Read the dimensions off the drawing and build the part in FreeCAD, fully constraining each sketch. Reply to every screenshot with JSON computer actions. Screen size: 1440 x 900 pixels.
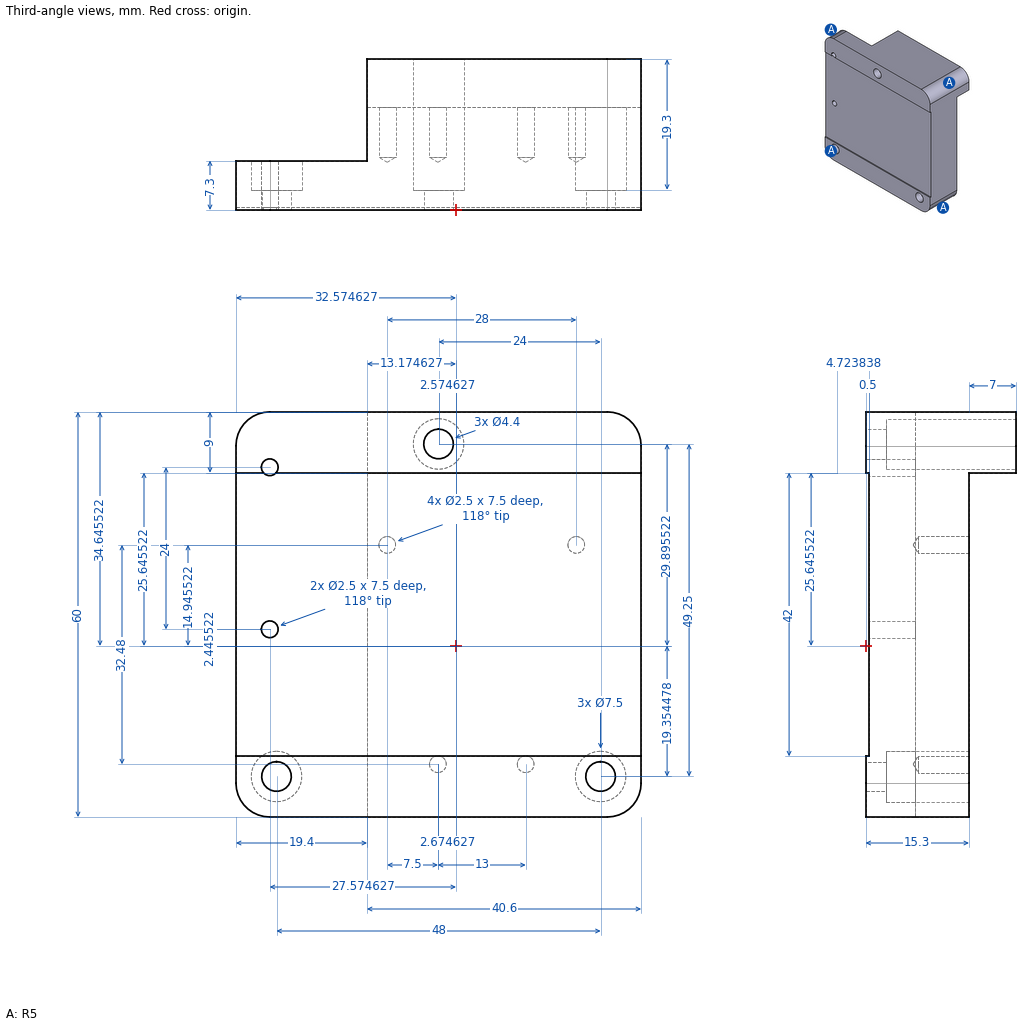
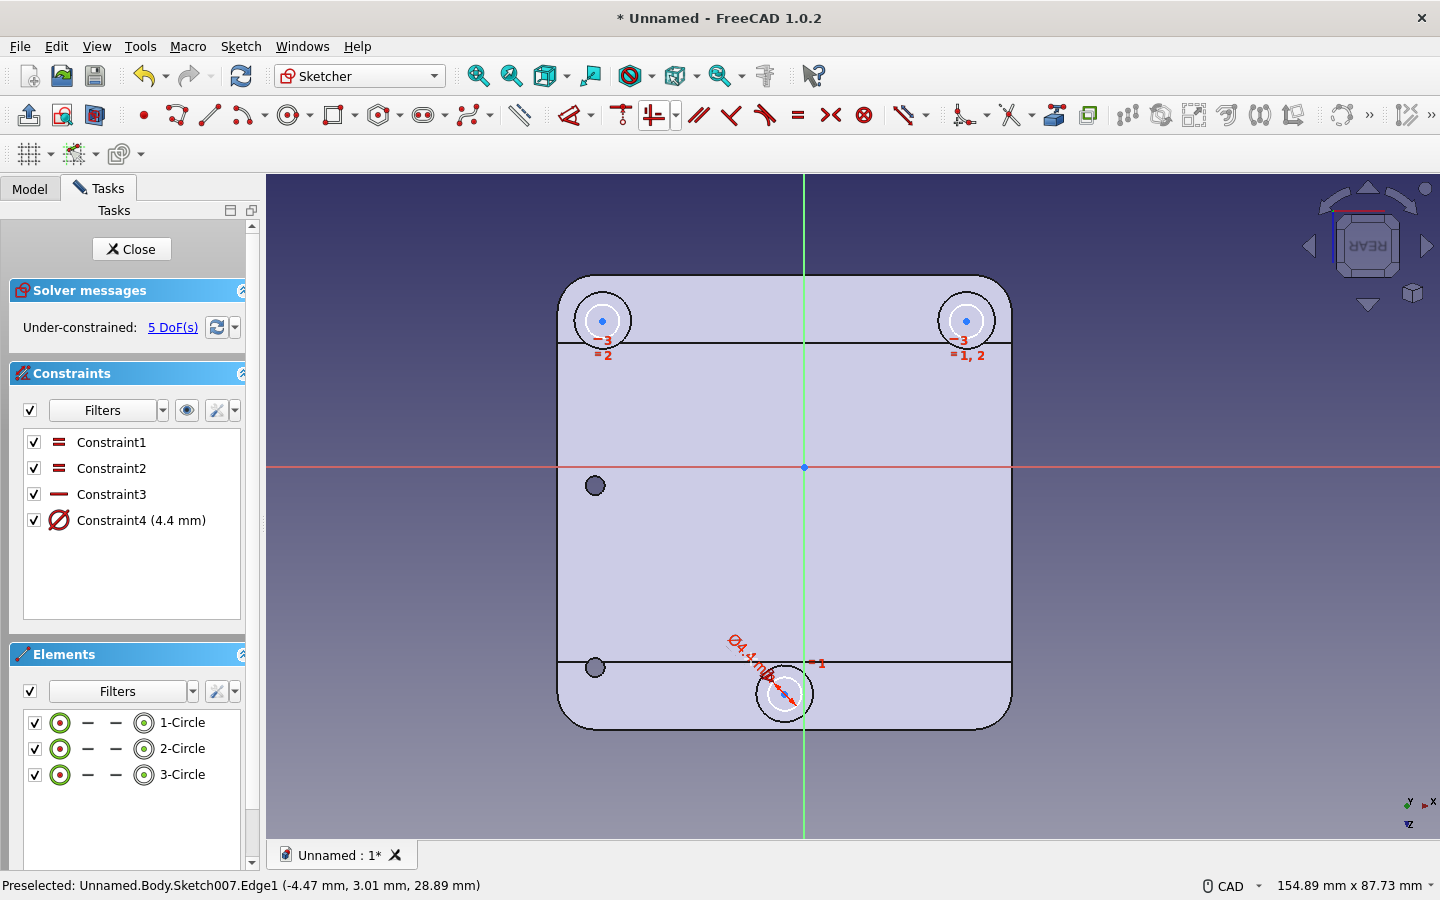
{"action": "left_click", "coordinate": [785, 694]}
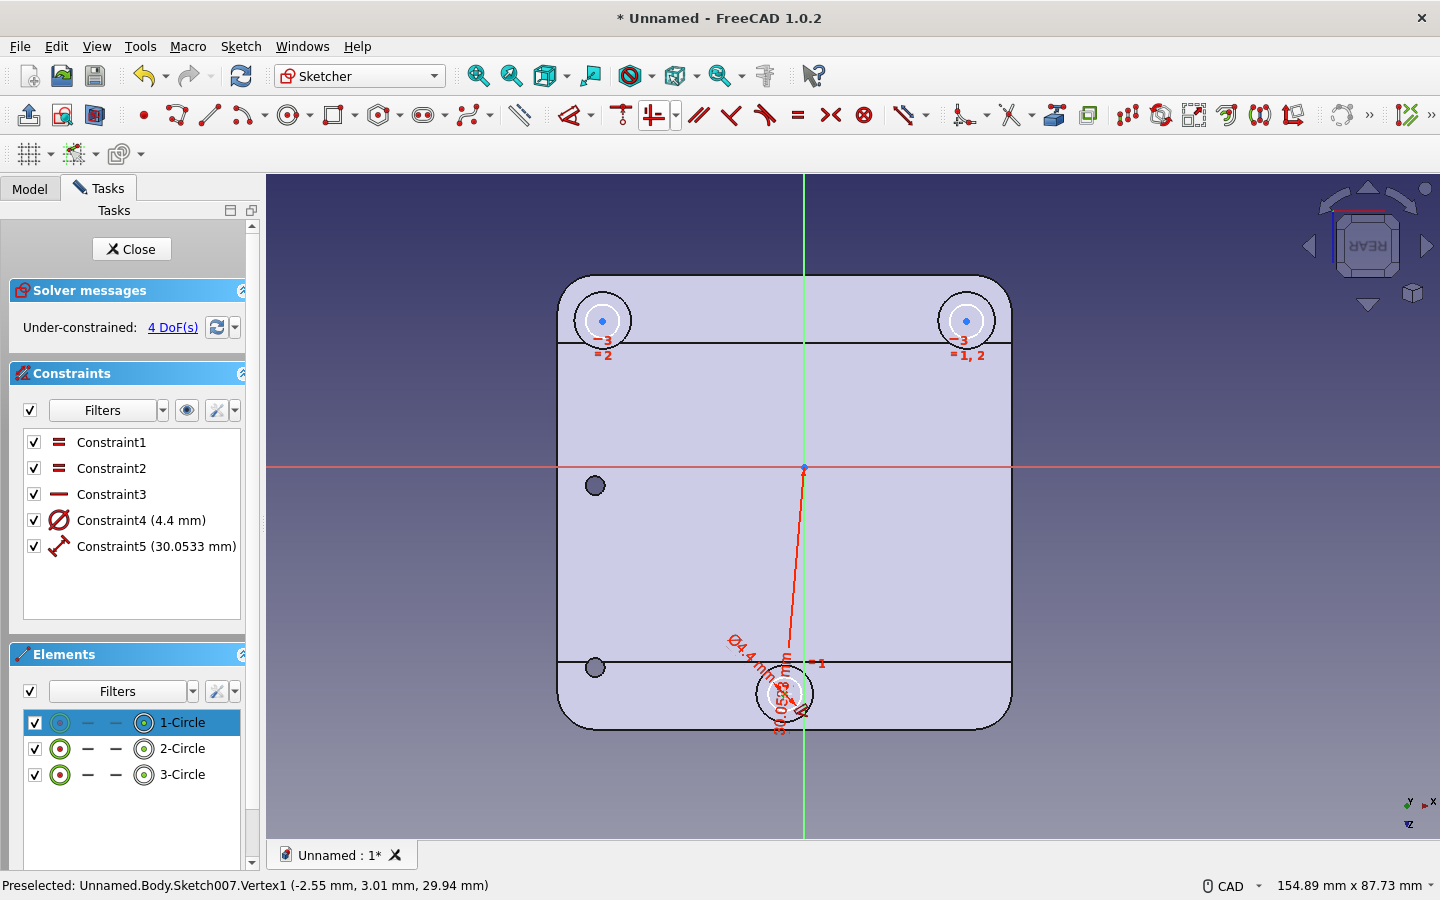
{"action": "left_click", "coordinate": [967, 321]}
{"action": "left_click", "coordinate": [876, 728]}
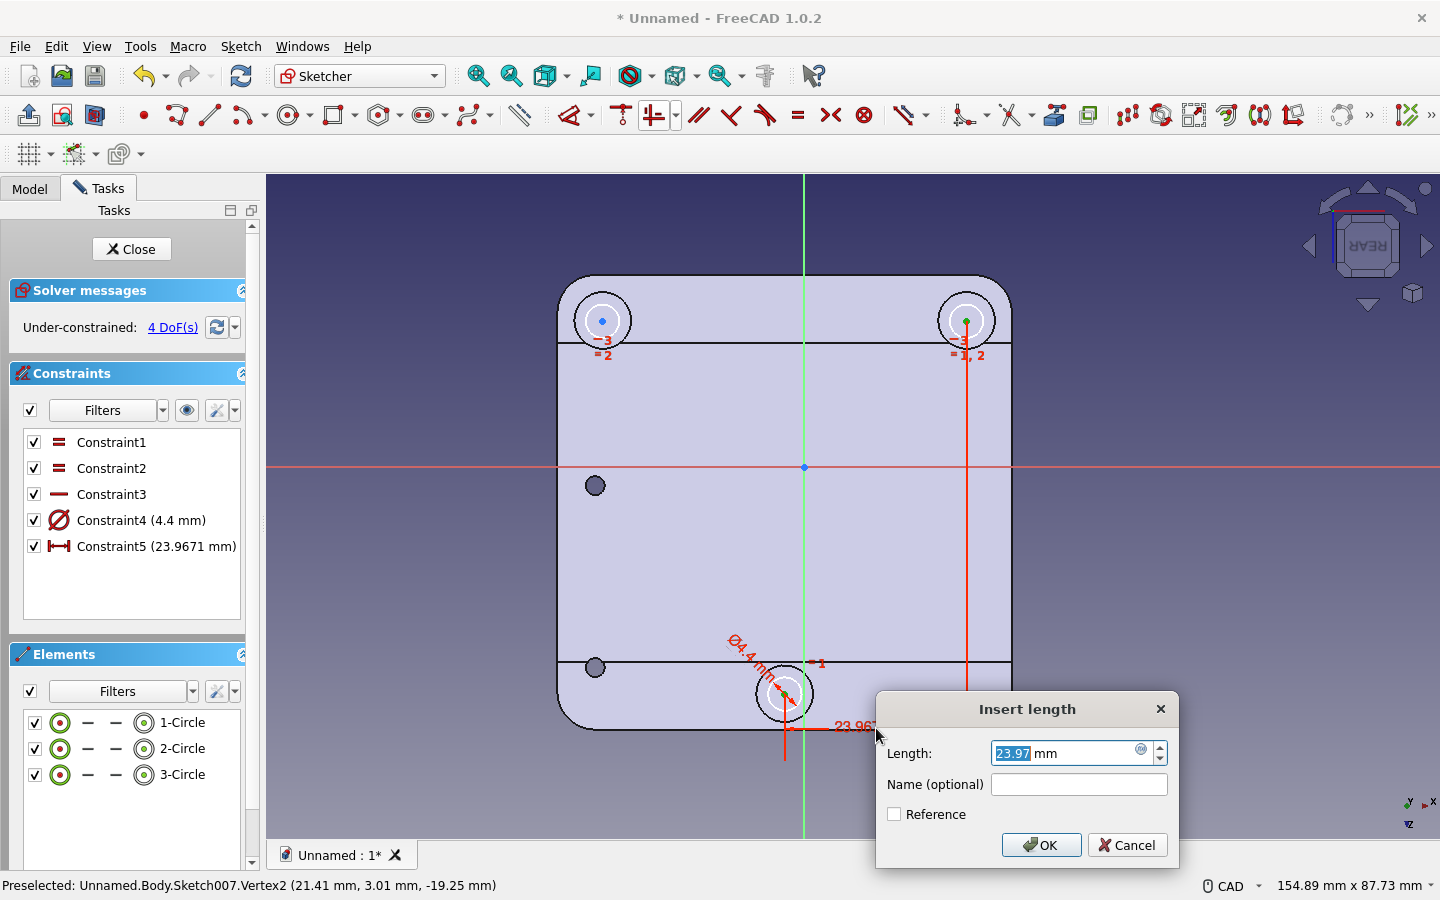
{"action": "type", "text": "24"}
{"action": "key", "text": "Return"}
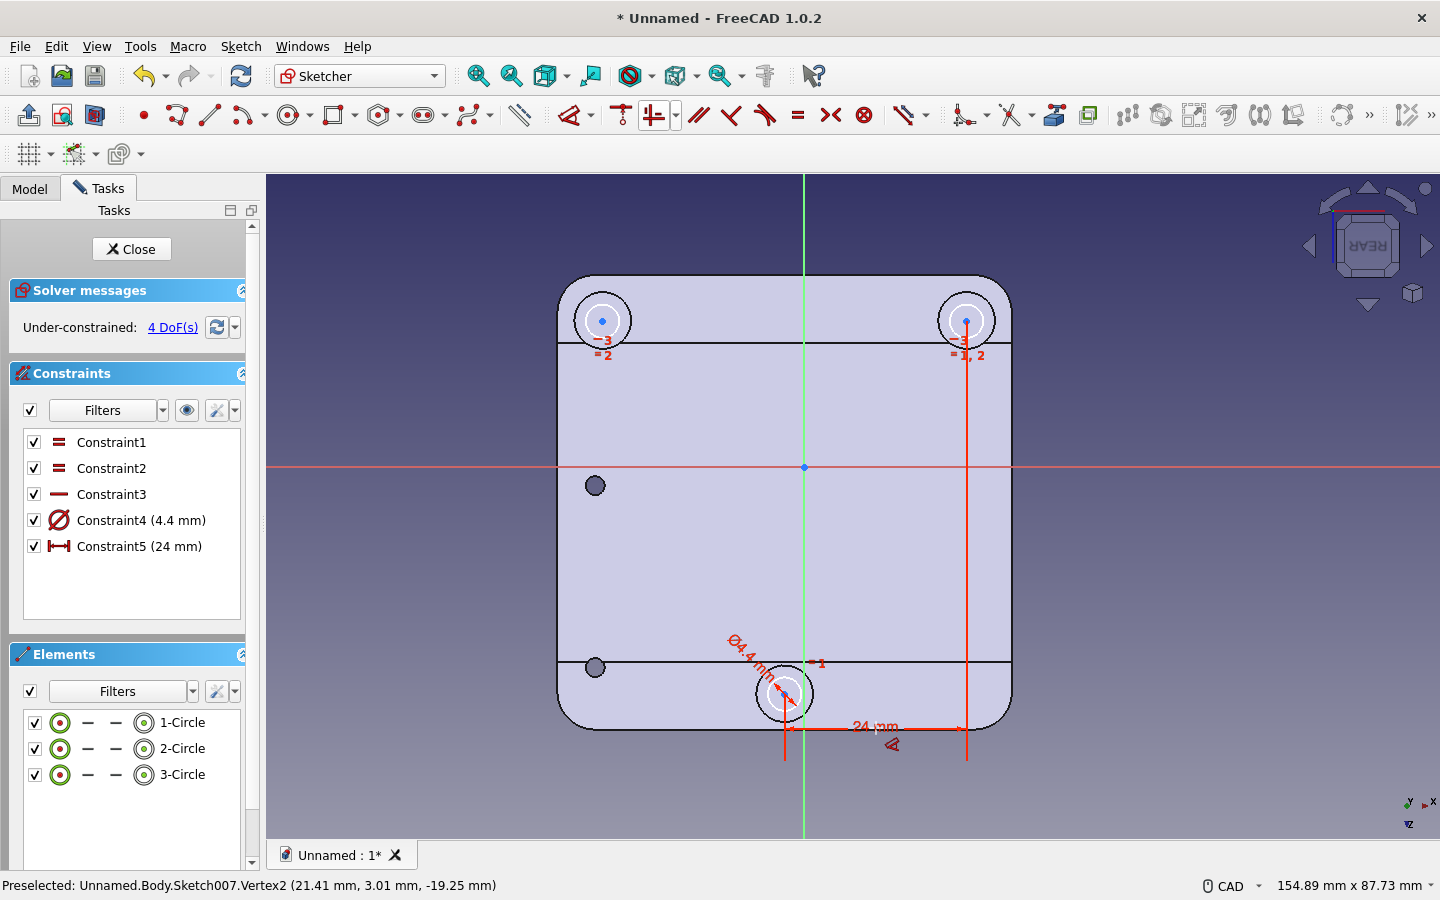
{"action": "left_click", "coordinate": [967, 321]}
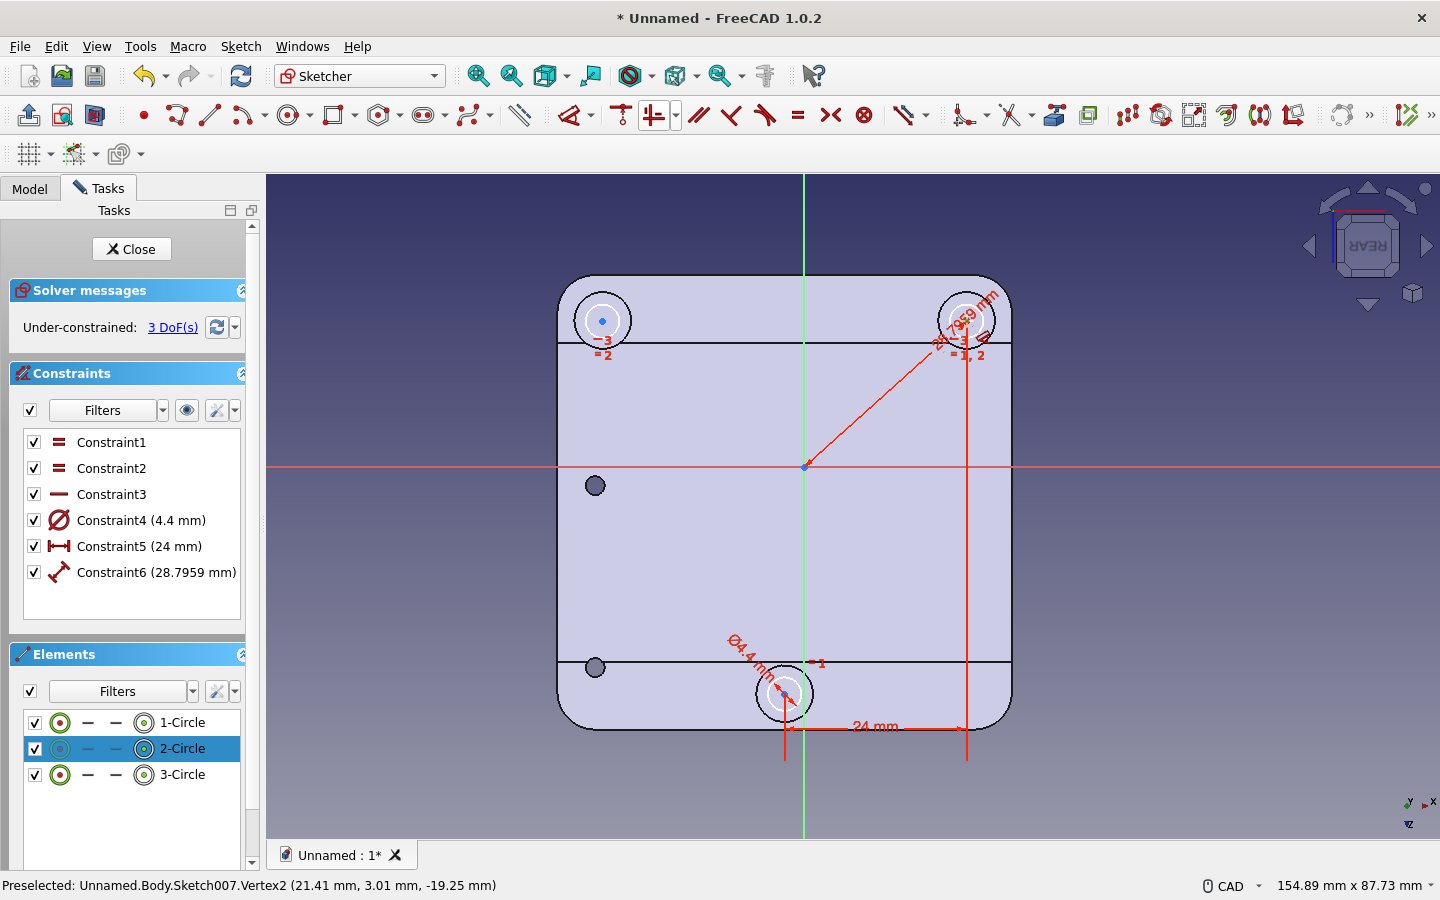
{"action": "left_click", "coordinate": [603, 321]}
{"action": "left_click", "coordinate": [785, 287]}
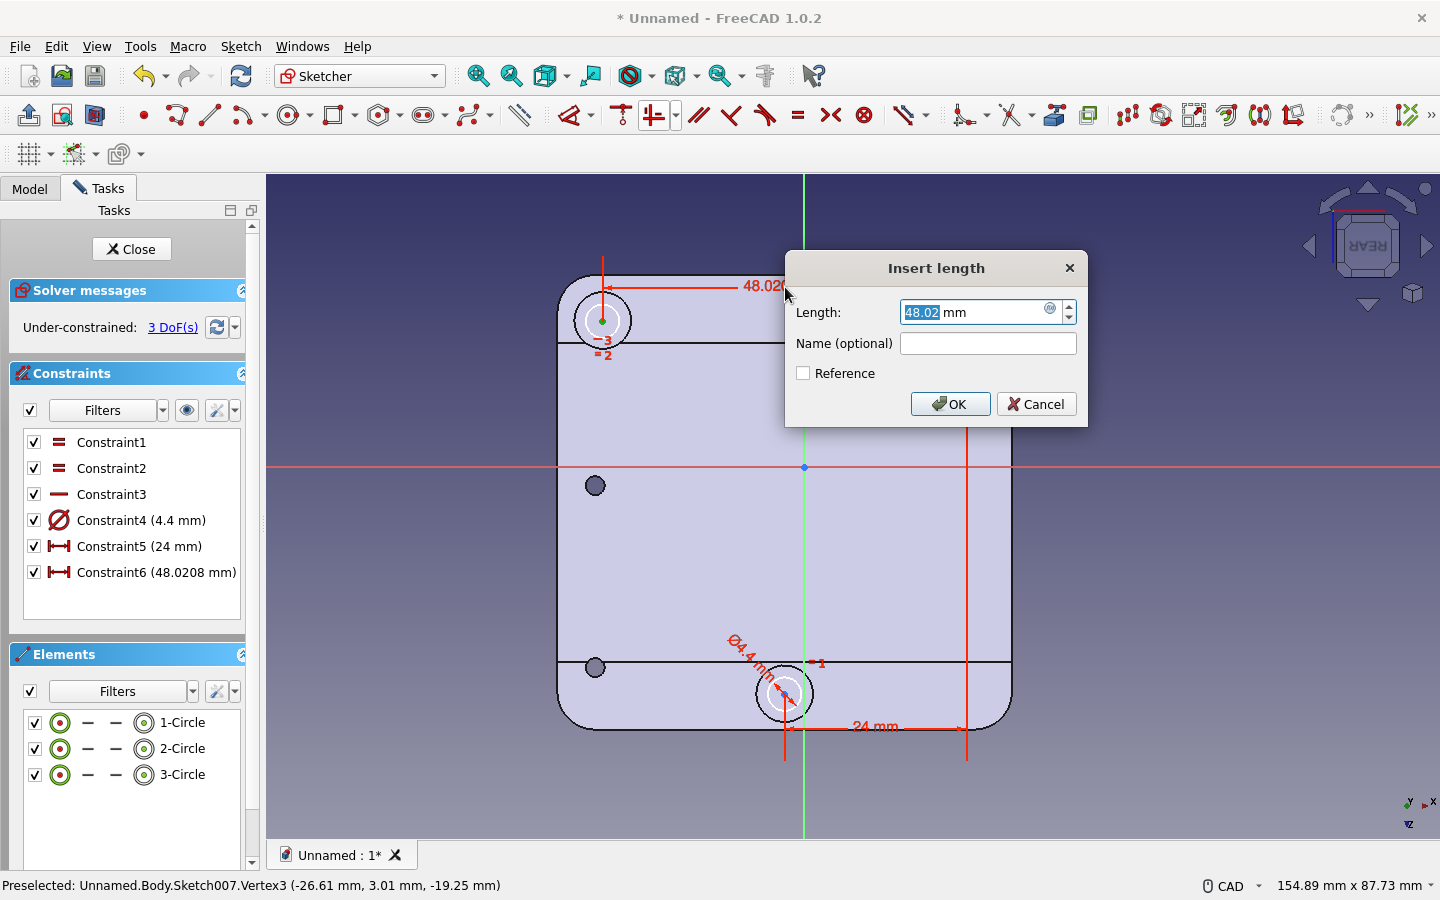
{"action": "type", "text": "48"}
{"action": "key", "text": "Return"}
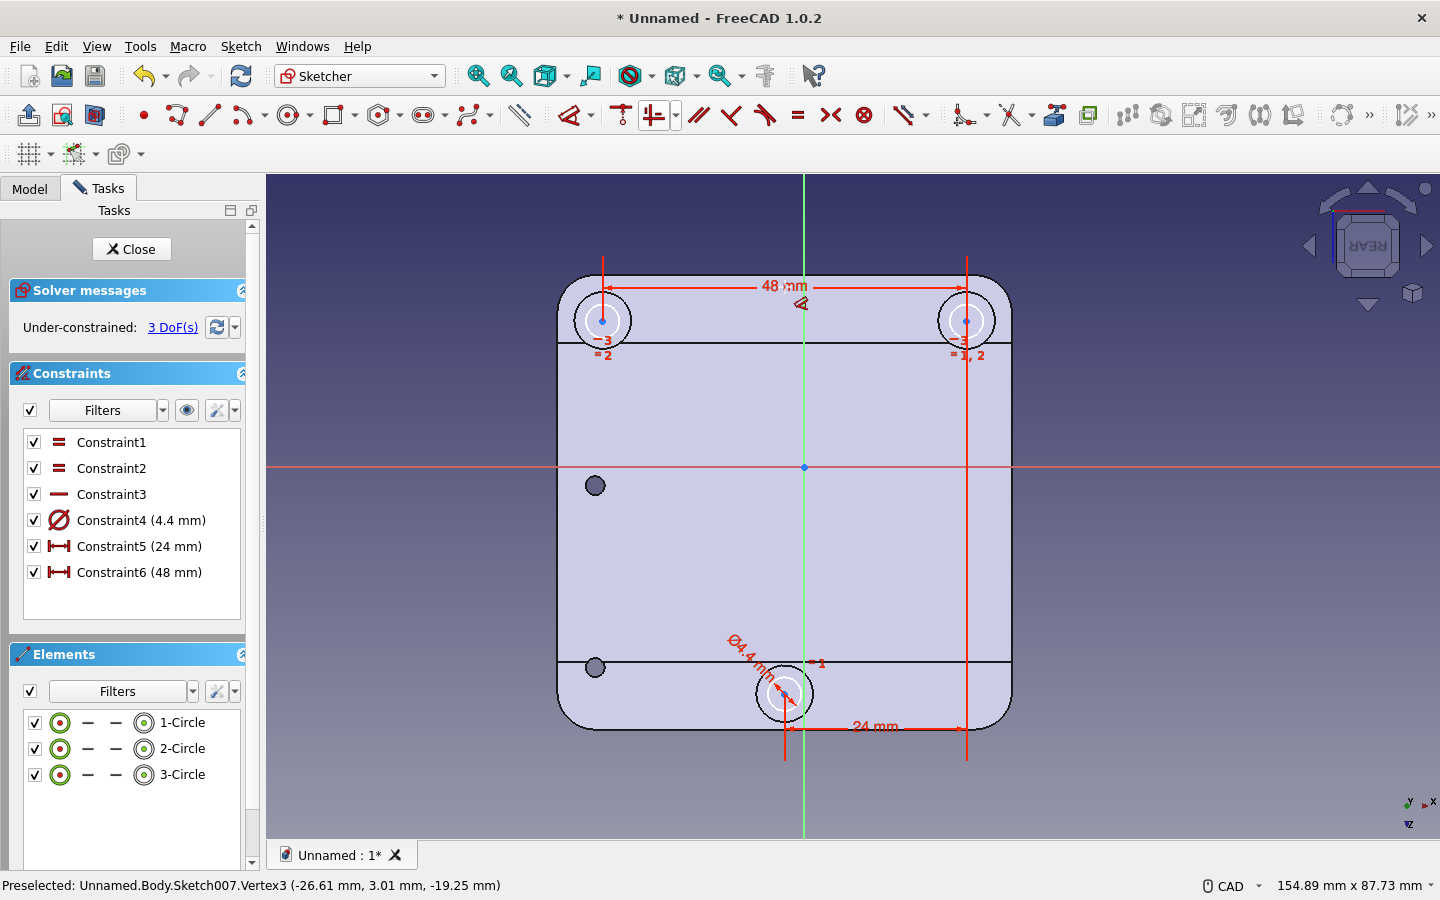
{"action": "left_click", "coordinate": [785, 694]}